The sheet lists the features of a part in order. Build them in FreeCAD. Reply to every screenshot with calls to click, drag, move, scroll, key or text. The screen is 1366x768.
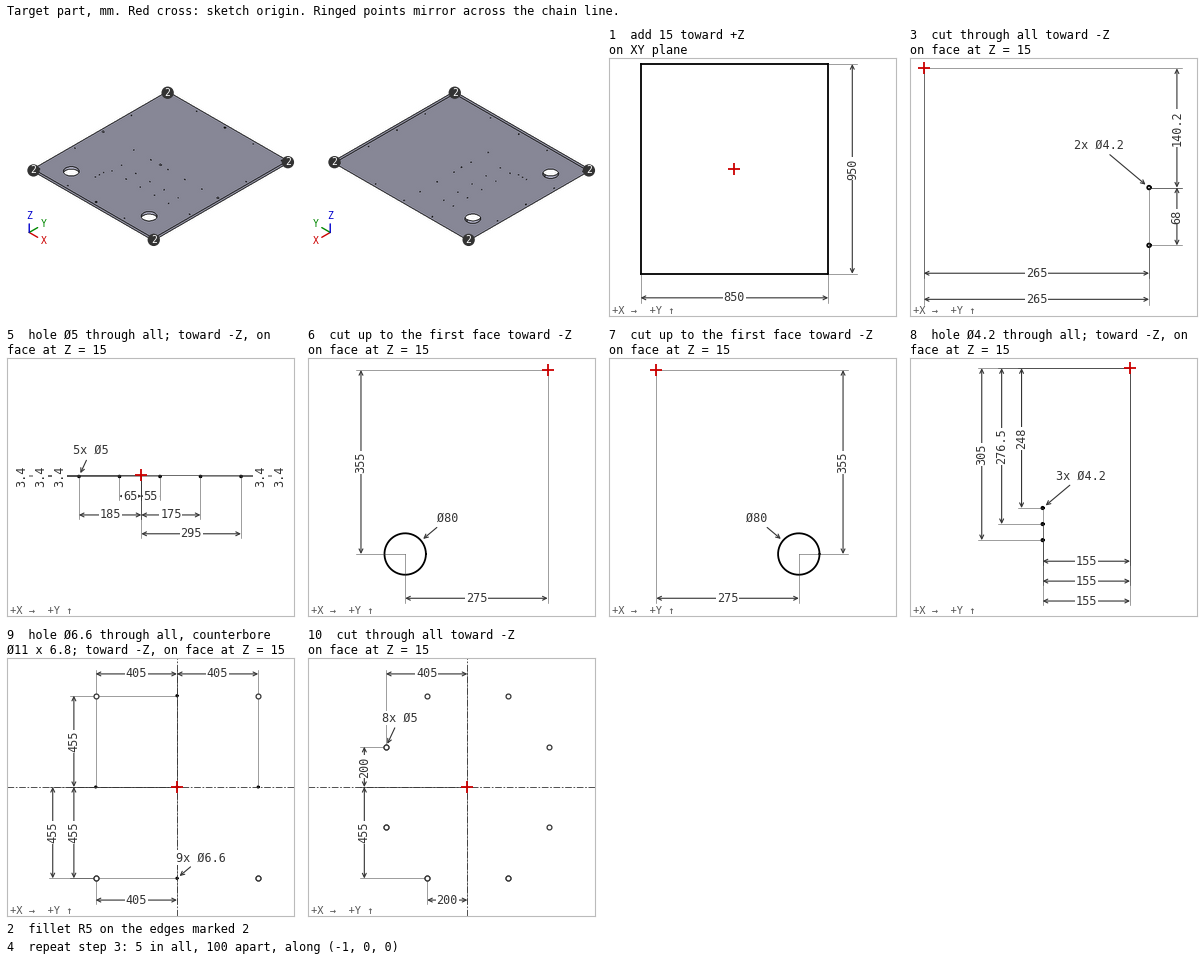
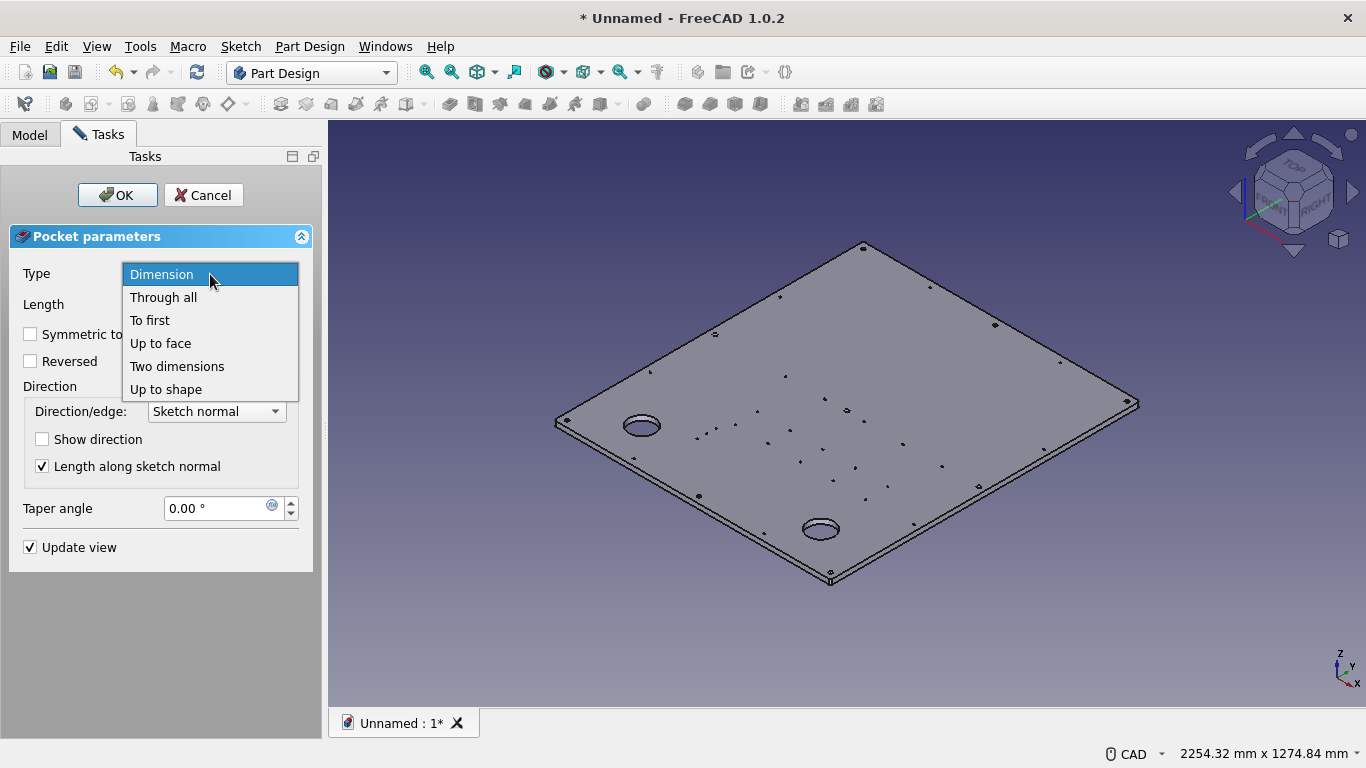
click(208, 298)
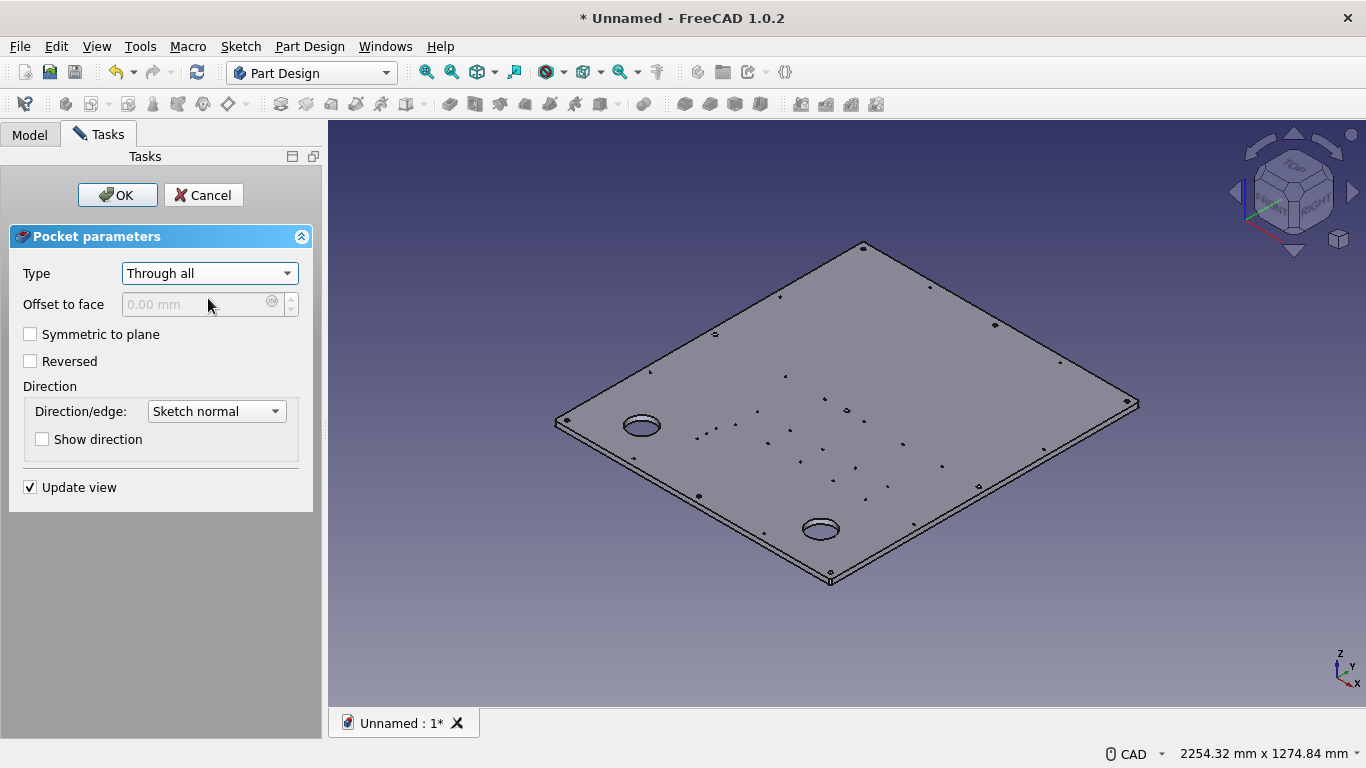
click(118, 195)